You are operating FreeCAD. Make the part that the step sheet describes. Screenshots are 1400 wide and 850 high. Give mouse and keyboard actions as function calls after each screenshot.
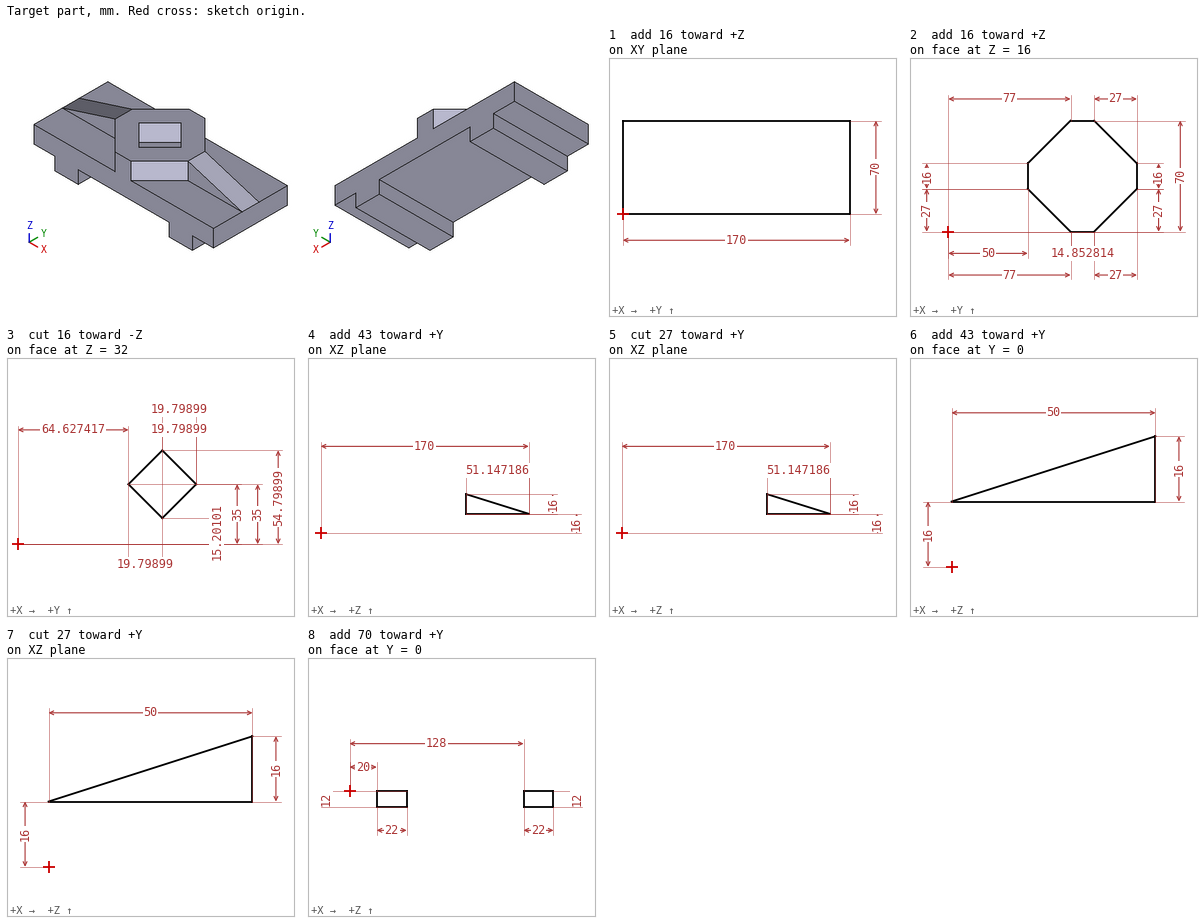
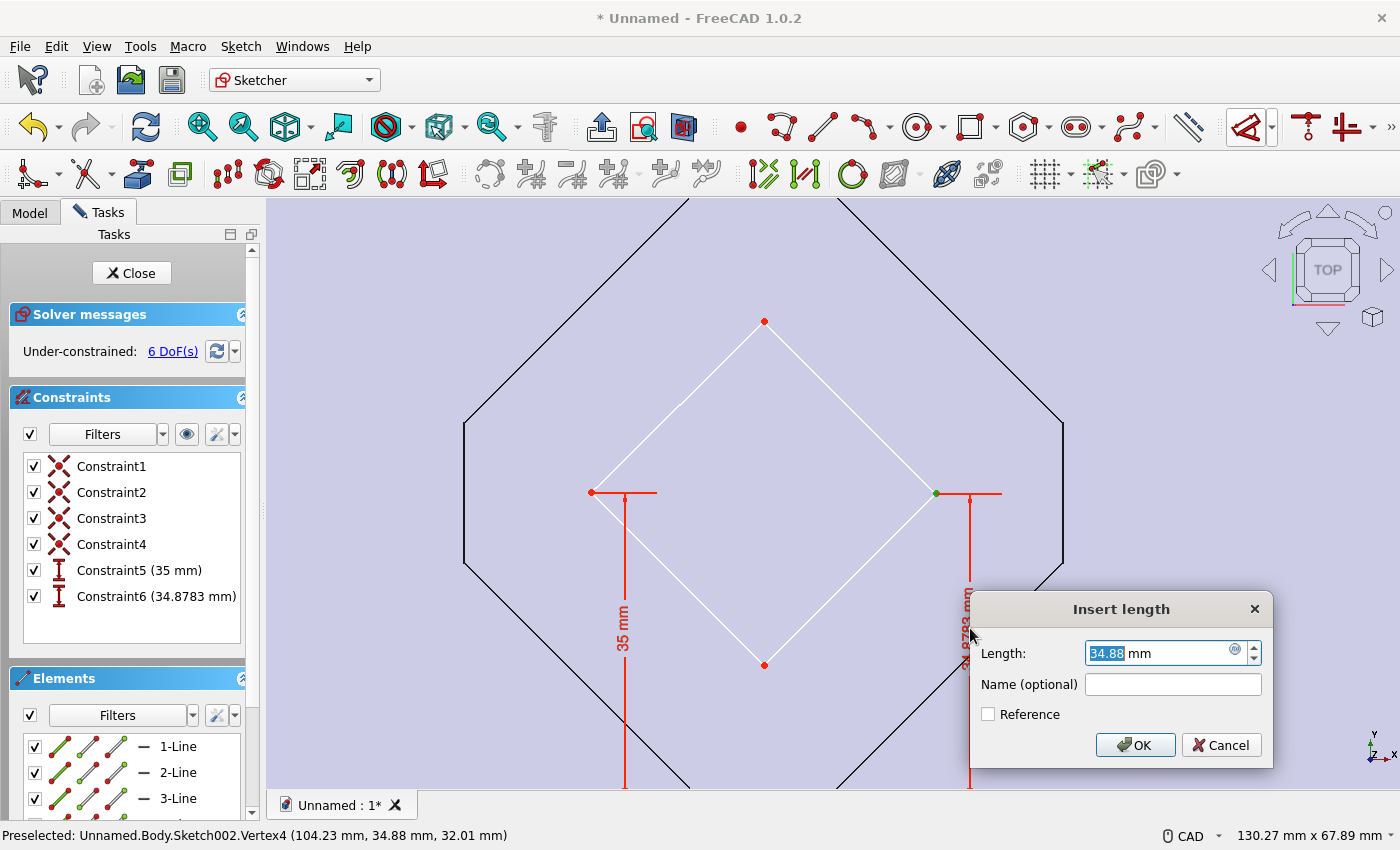
text(35)
key(Return)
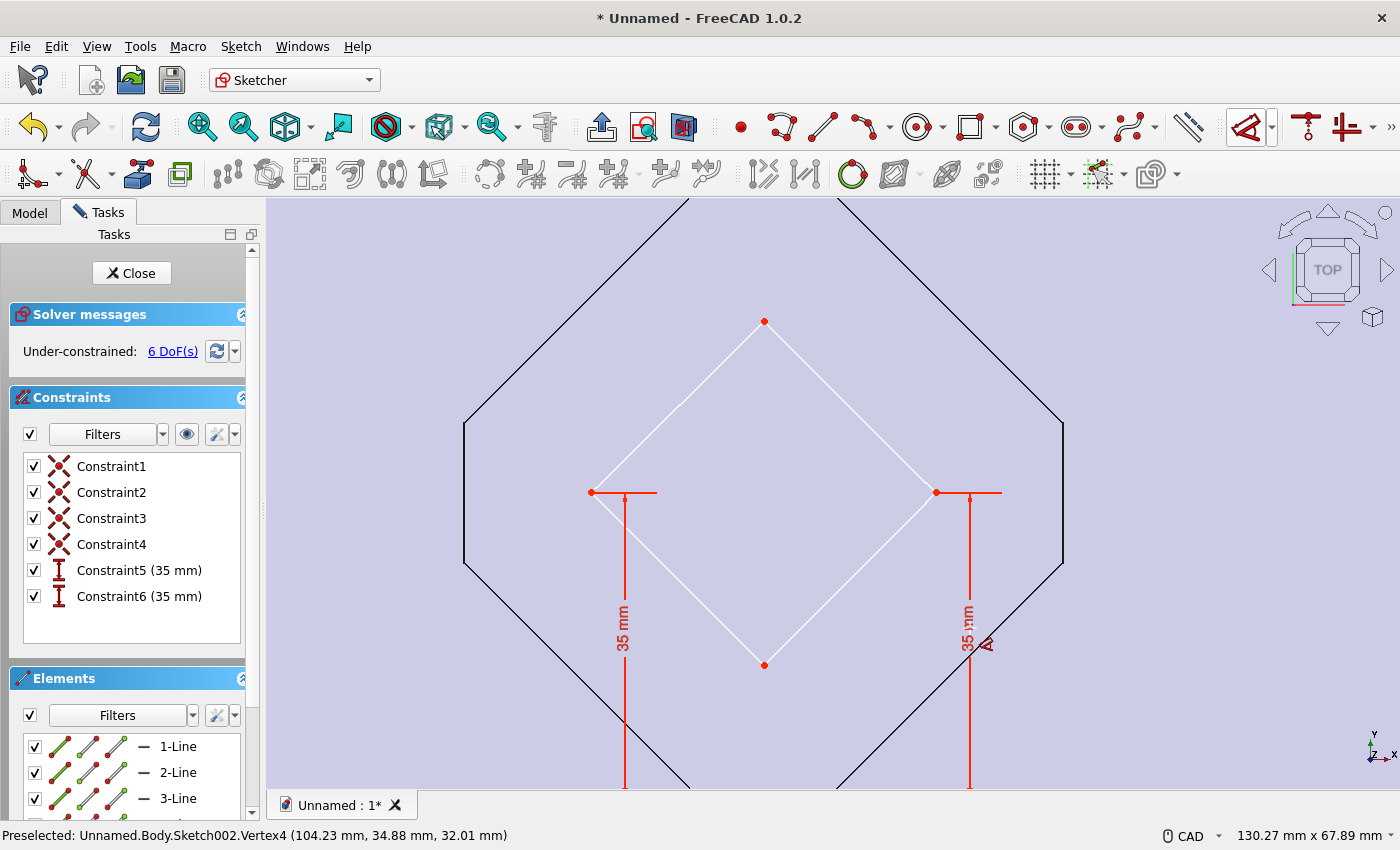
click(764, 666)
click(798, 714)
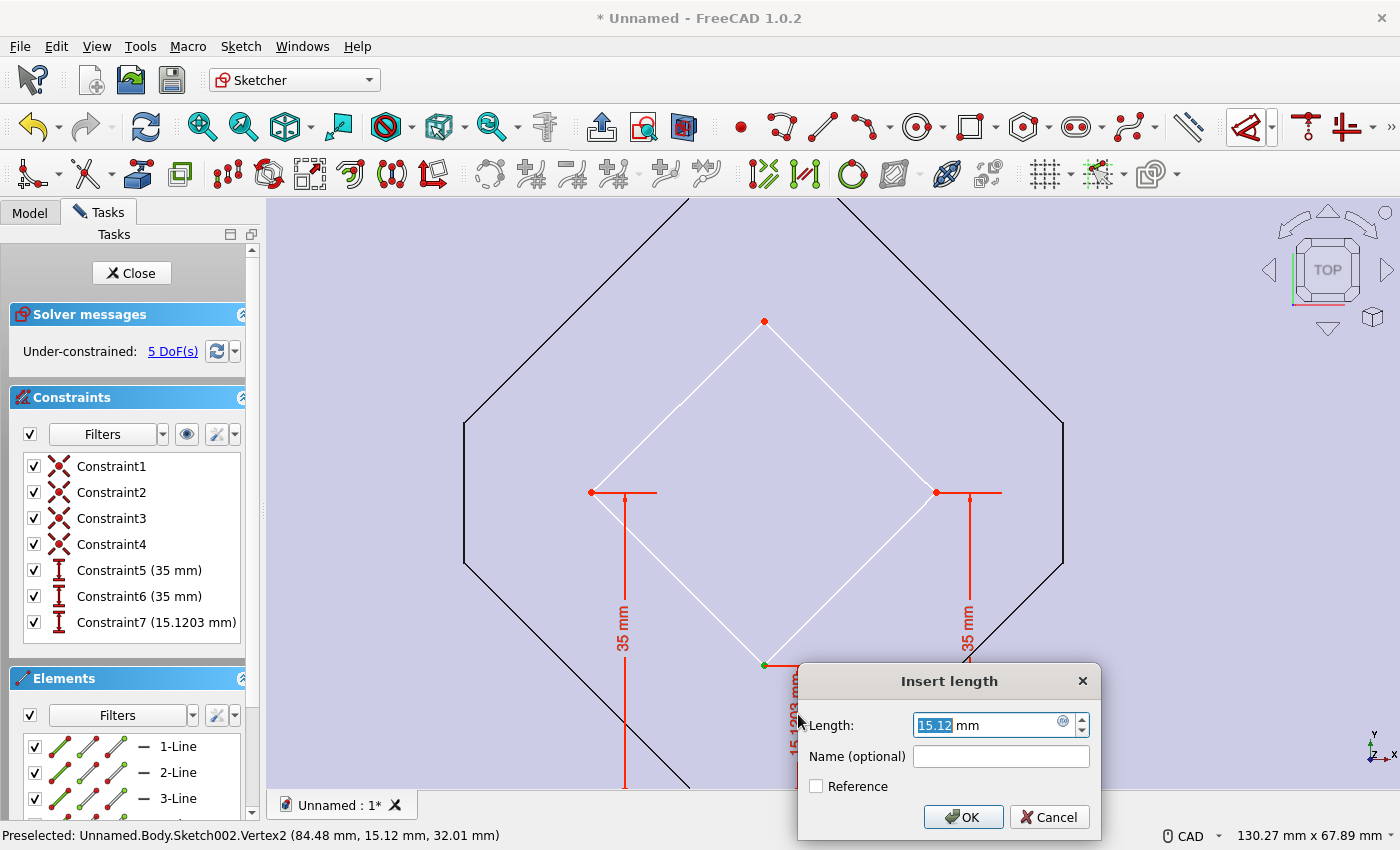
text(15.20101)
key(Return)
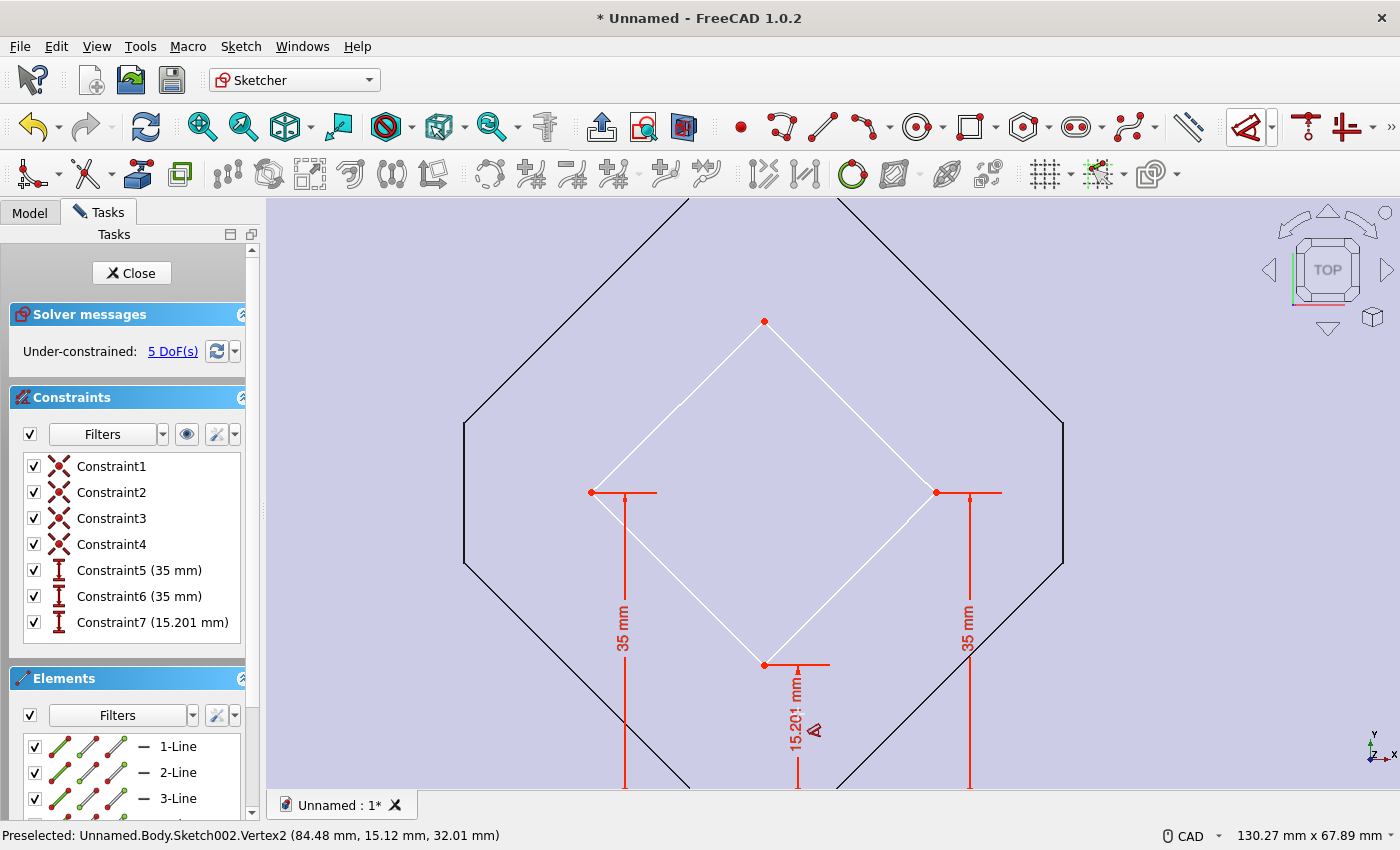
click(764, 322)
click(798, 542)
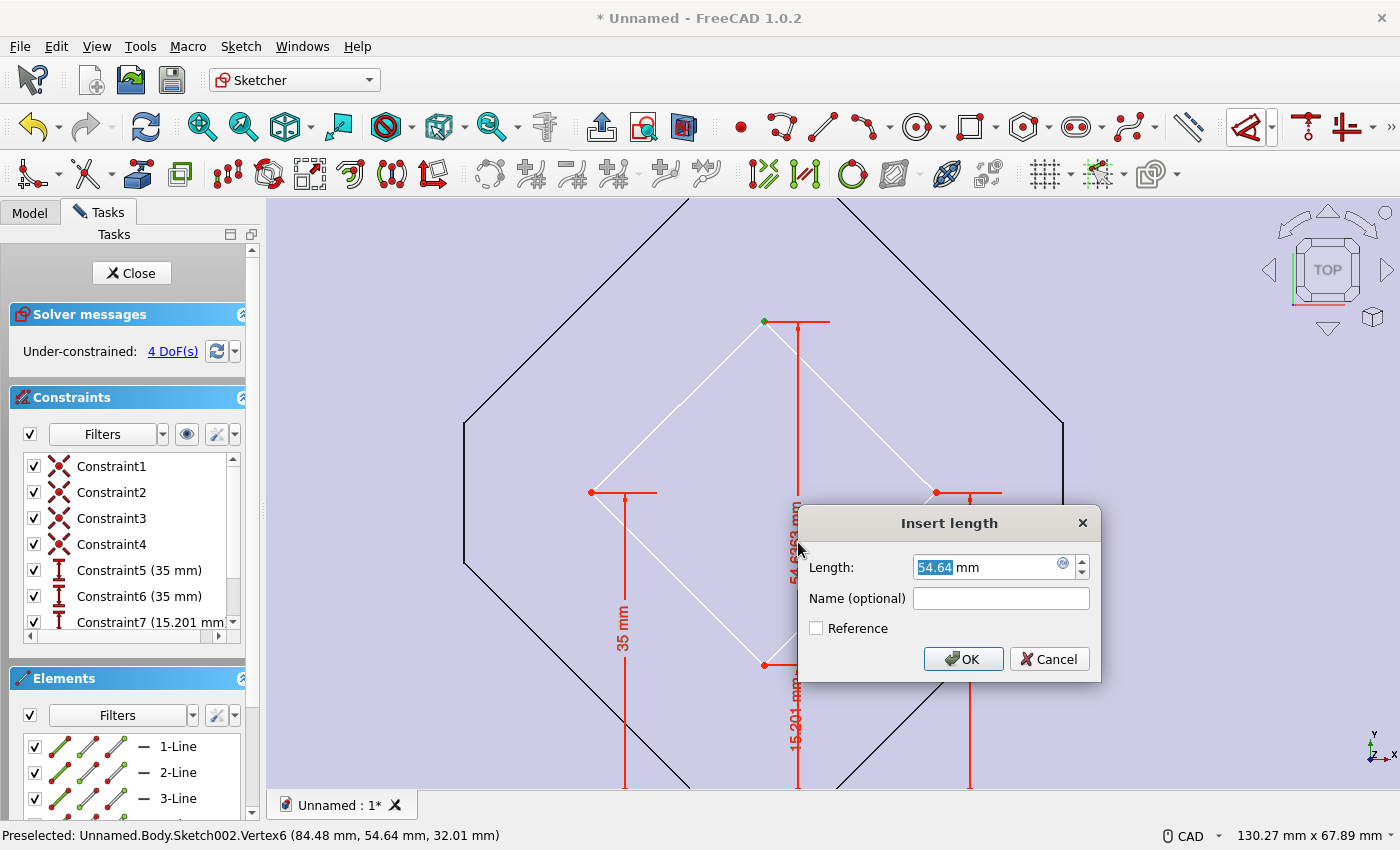
text(54.79899)
key(Return)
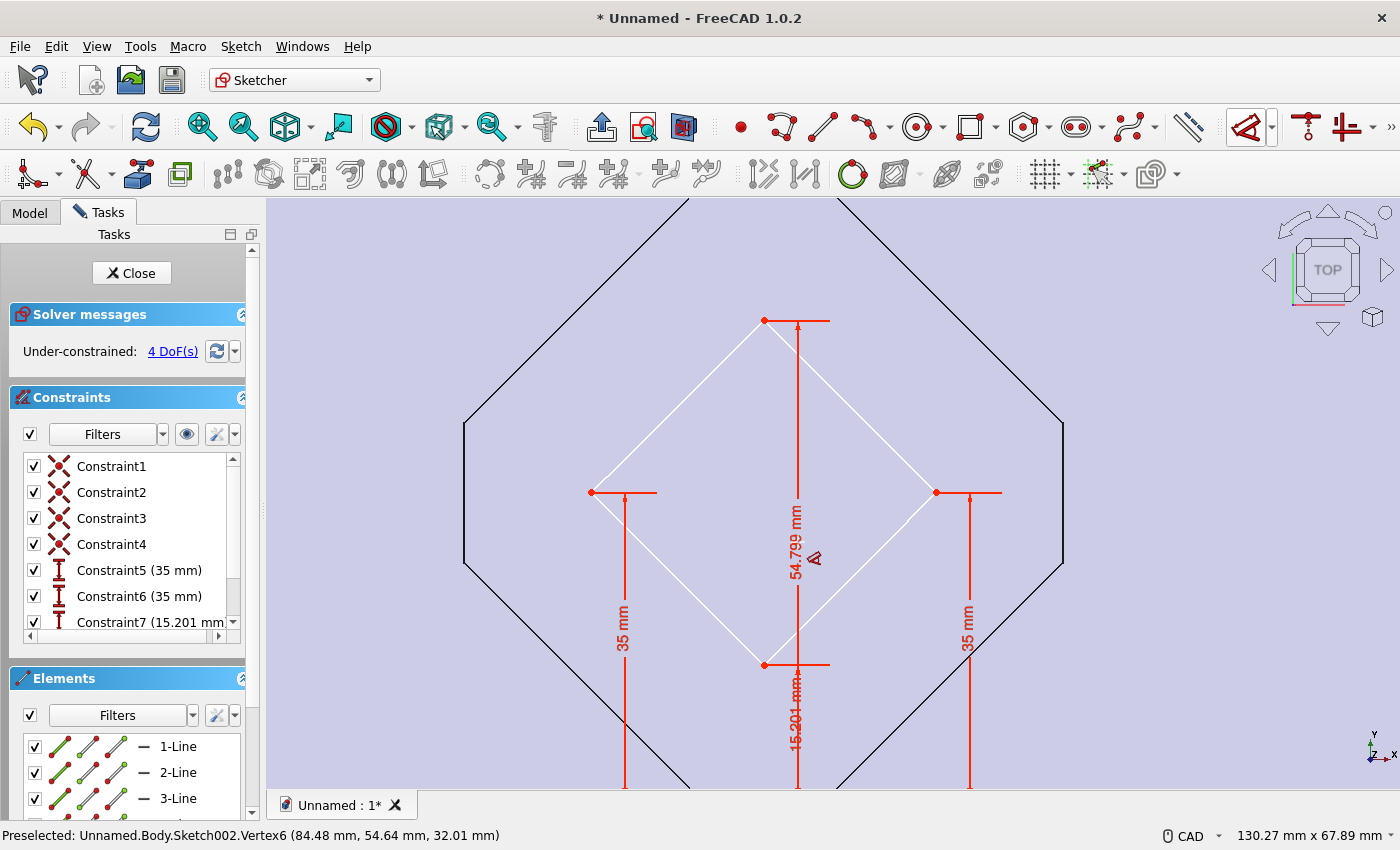
click(643, 545)
click(677, 699)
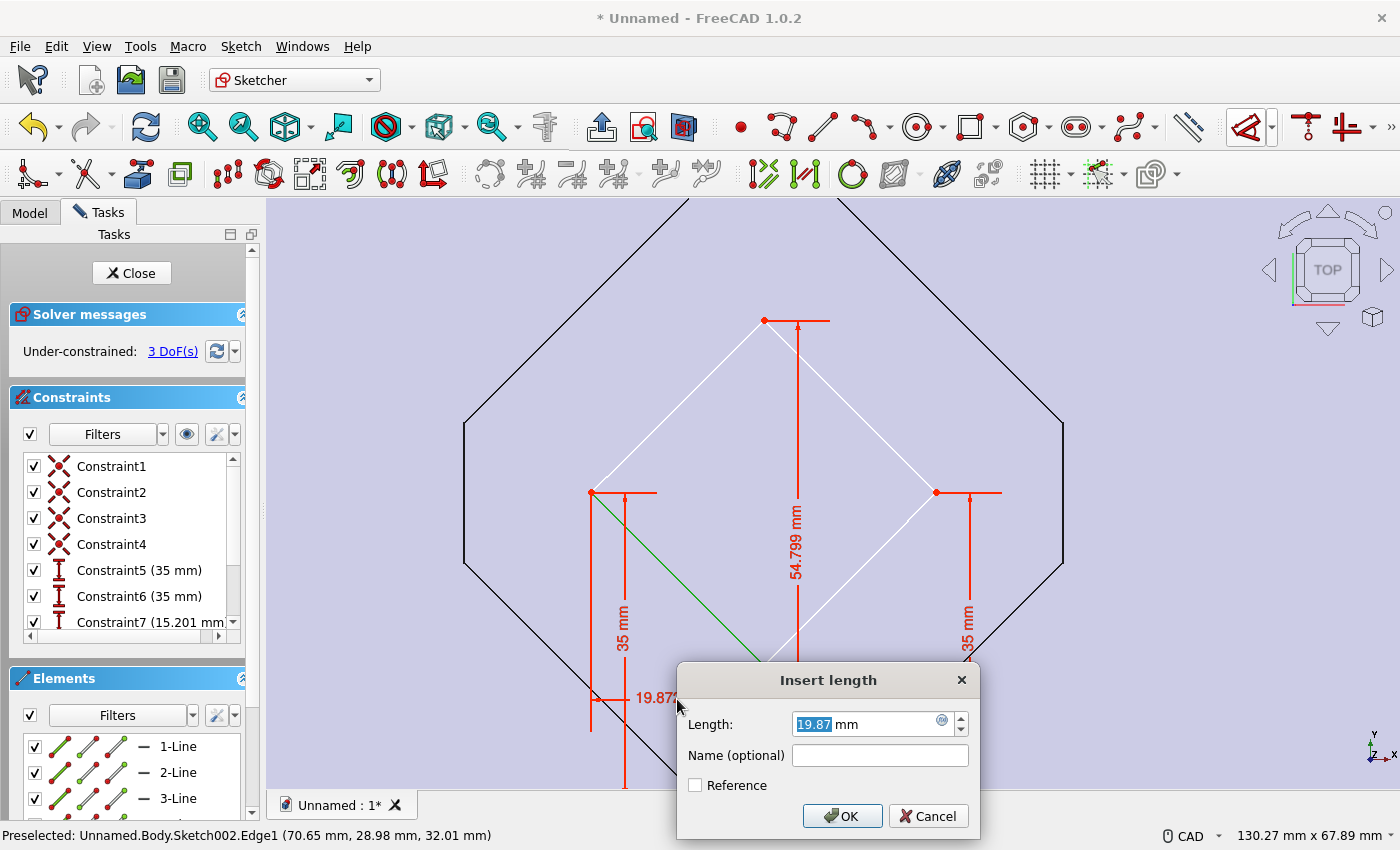
text(19.79899)
key(Return)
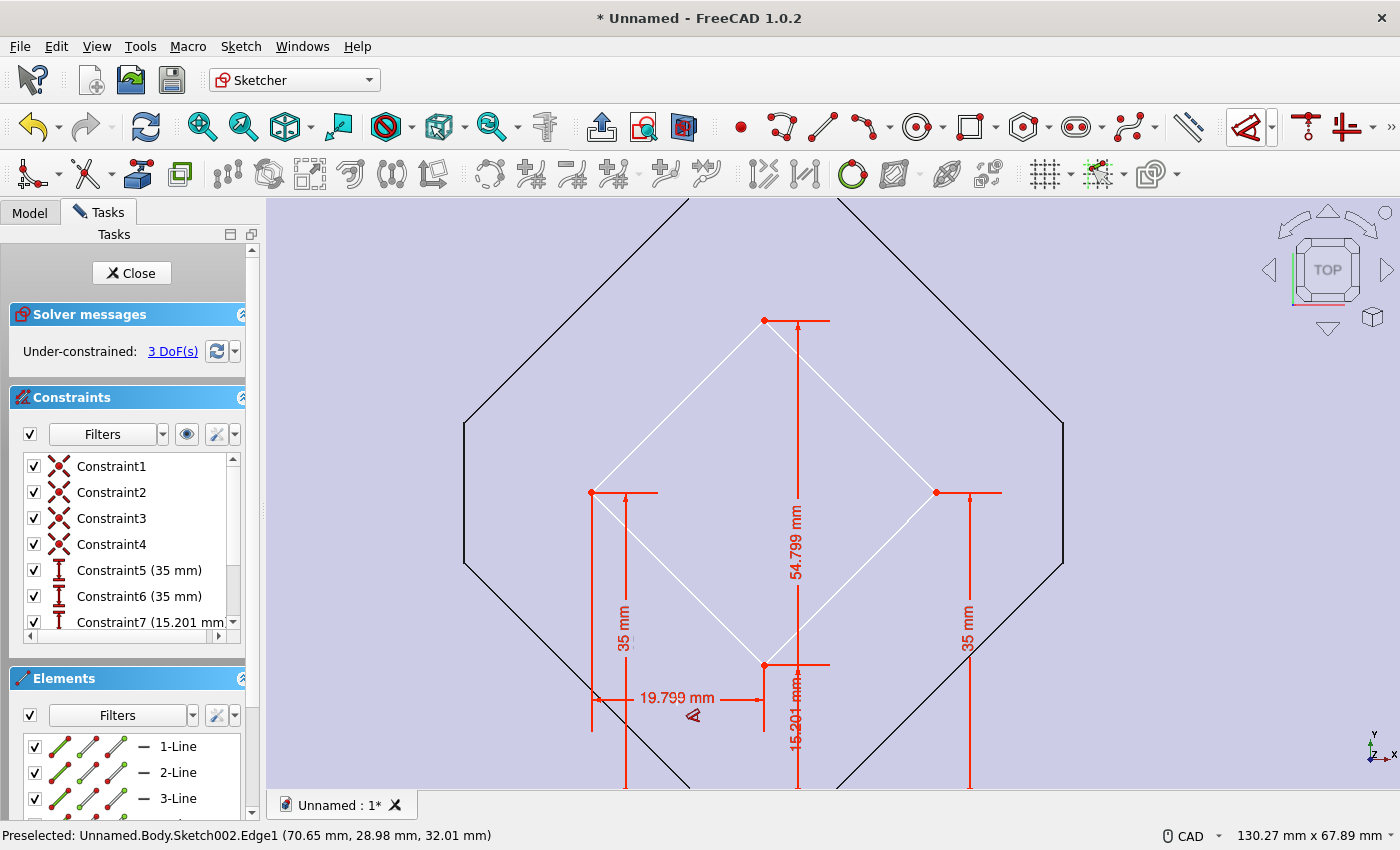
click(816, 614)
click(890, 699)